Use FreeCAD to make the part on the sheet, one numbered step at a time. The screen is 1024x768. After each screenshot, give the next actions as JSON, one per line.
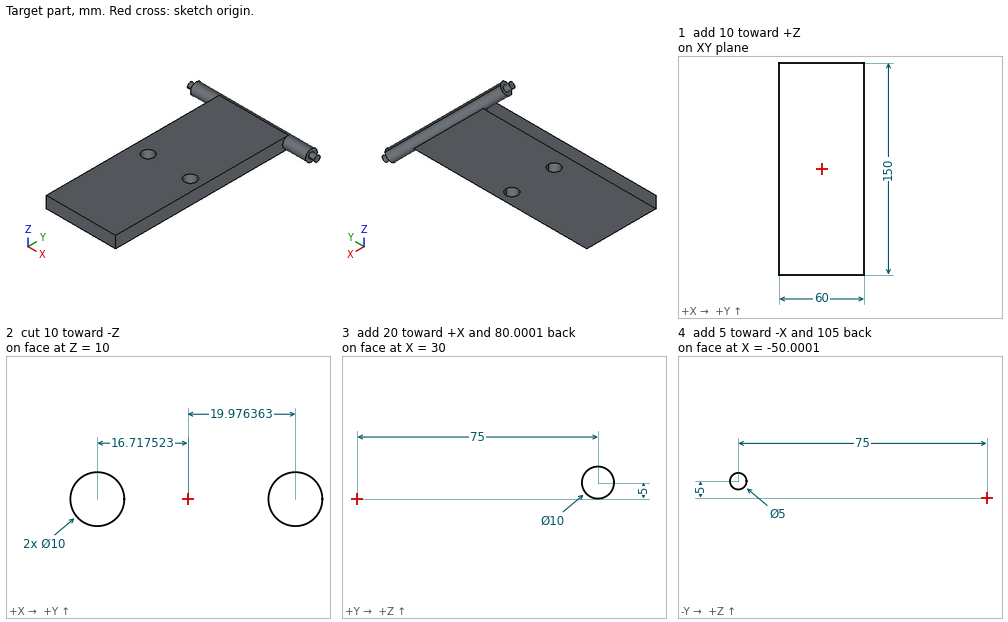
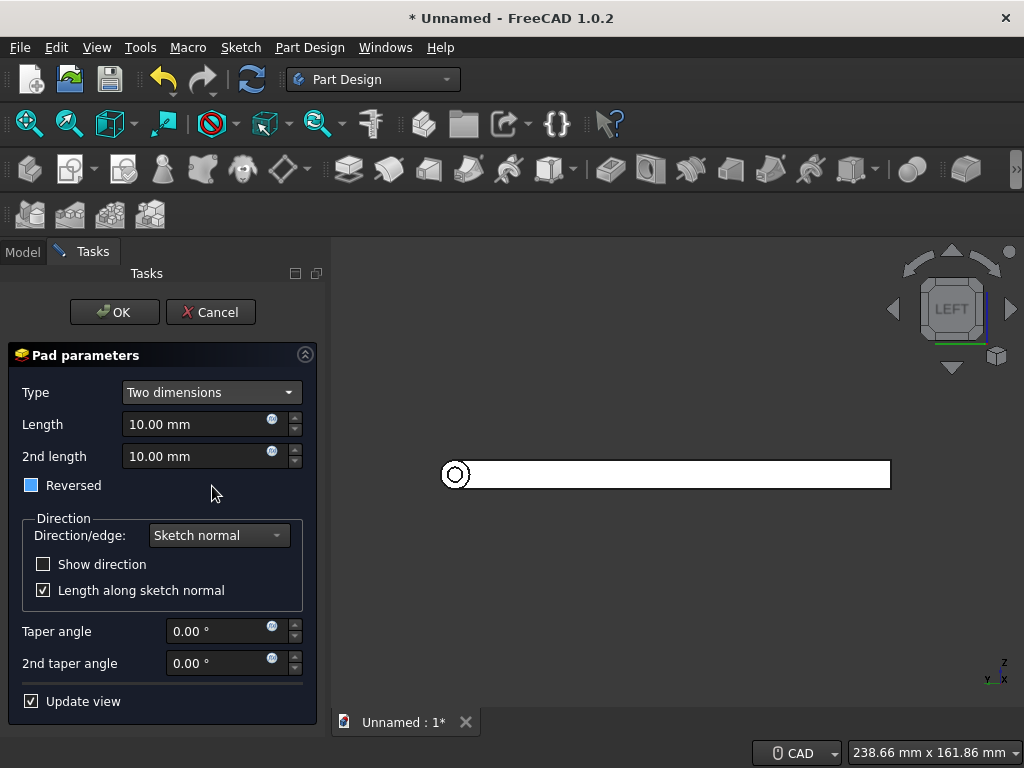
{"action": "triple_click", "coordinate": [204, 424]}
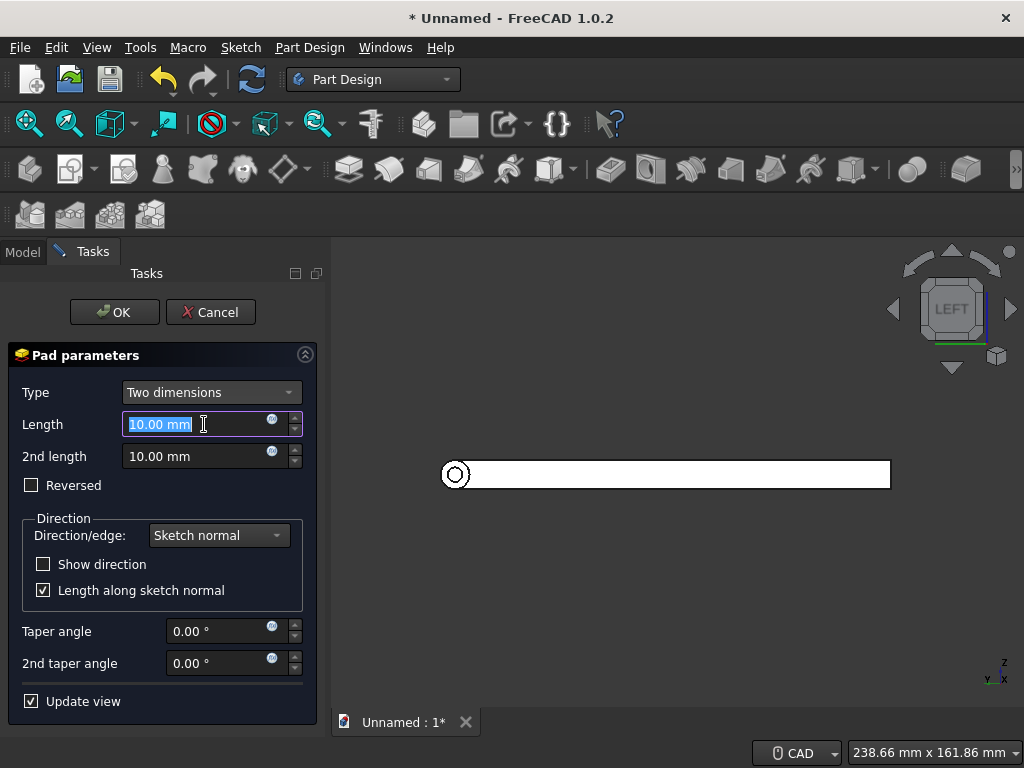
{"action": "type", "text": "5"}
{"action": "key", "text": "Tab"}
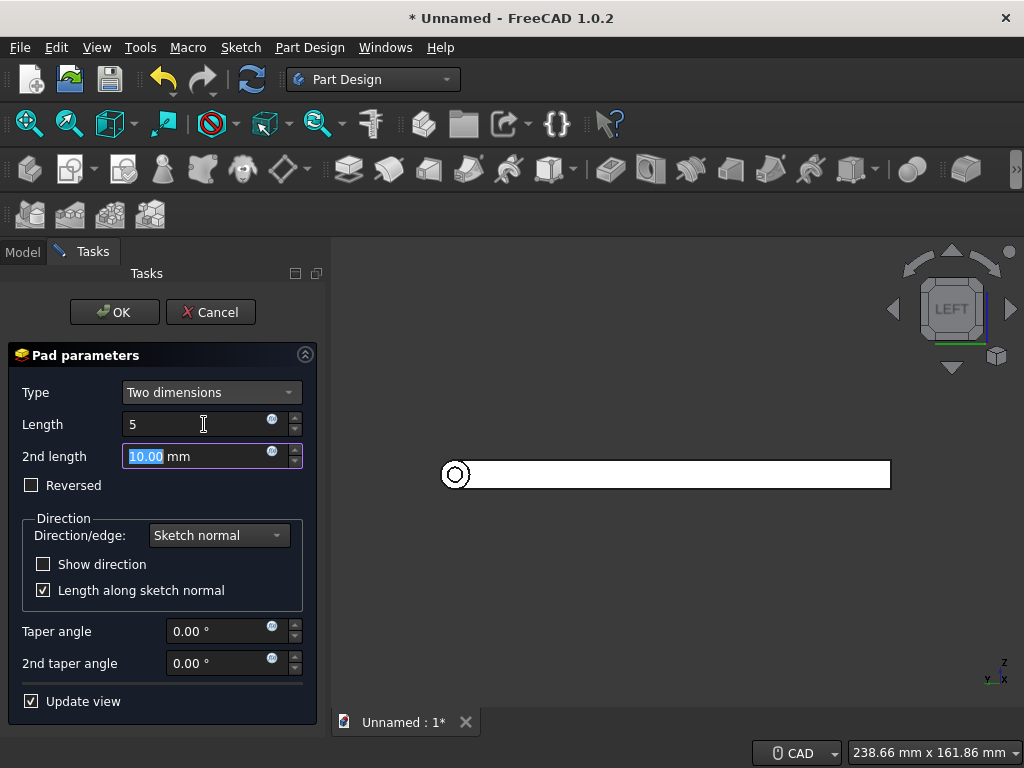
{"action": "type", "text": "105"}
{"action": "key", "text": "Tab"}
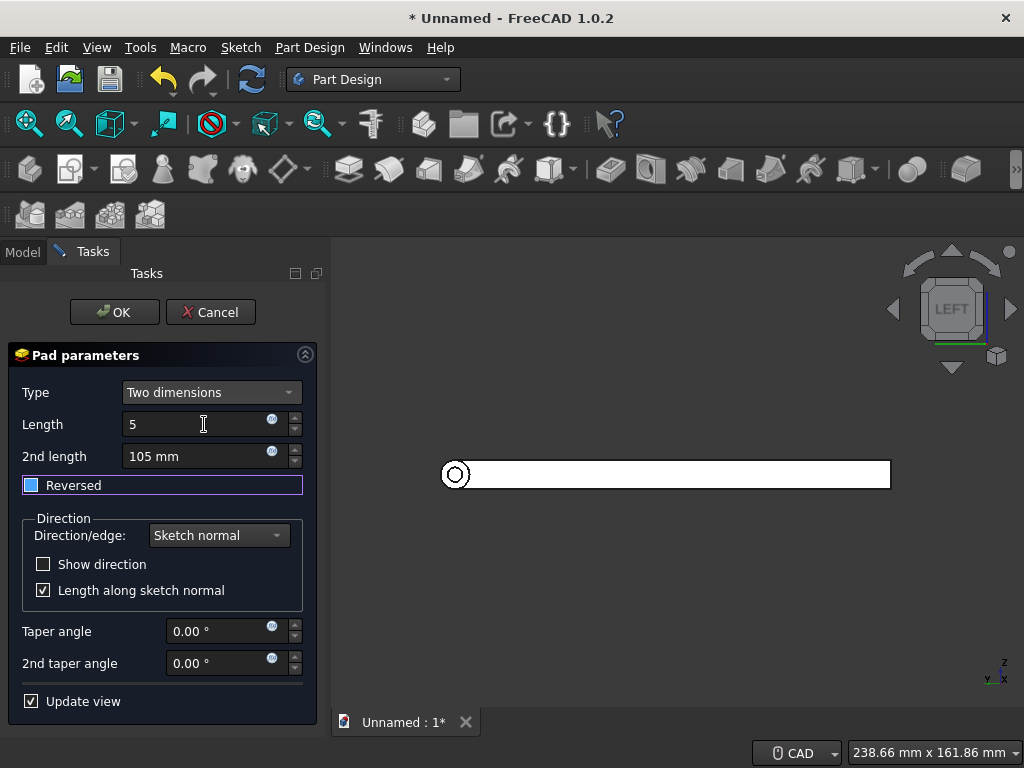
{"action": "left_click", "coordinate": [115, 312]}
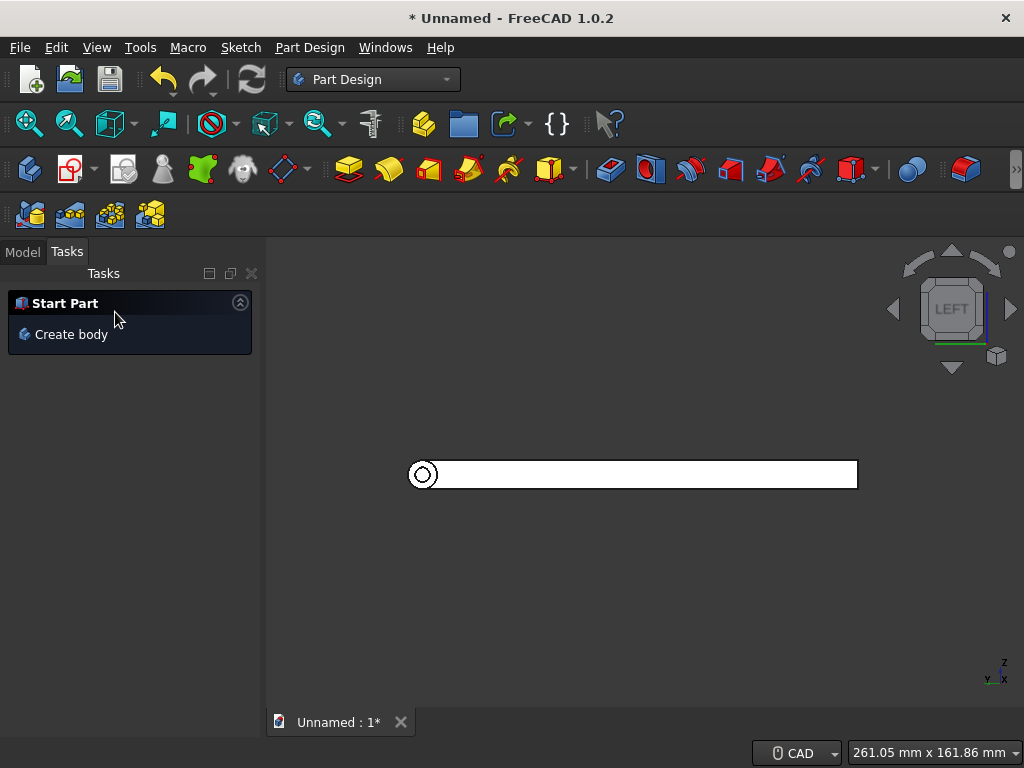
{"action": "key", "text": "0"}